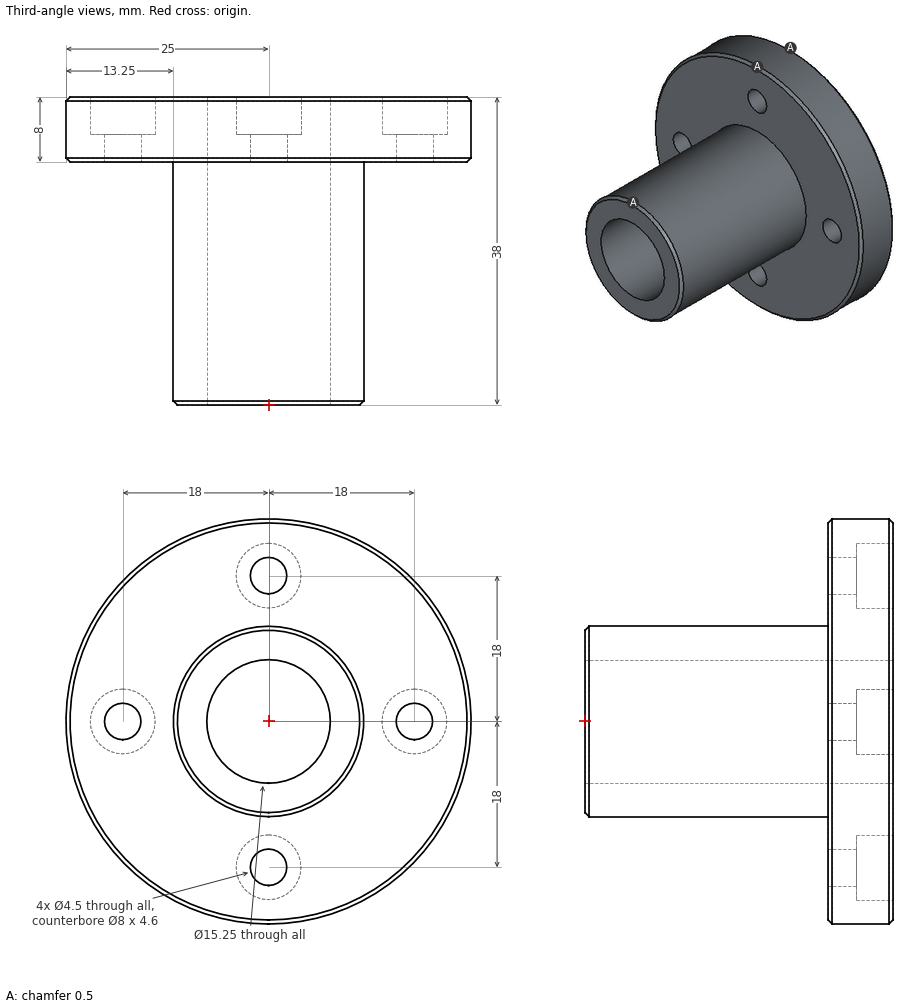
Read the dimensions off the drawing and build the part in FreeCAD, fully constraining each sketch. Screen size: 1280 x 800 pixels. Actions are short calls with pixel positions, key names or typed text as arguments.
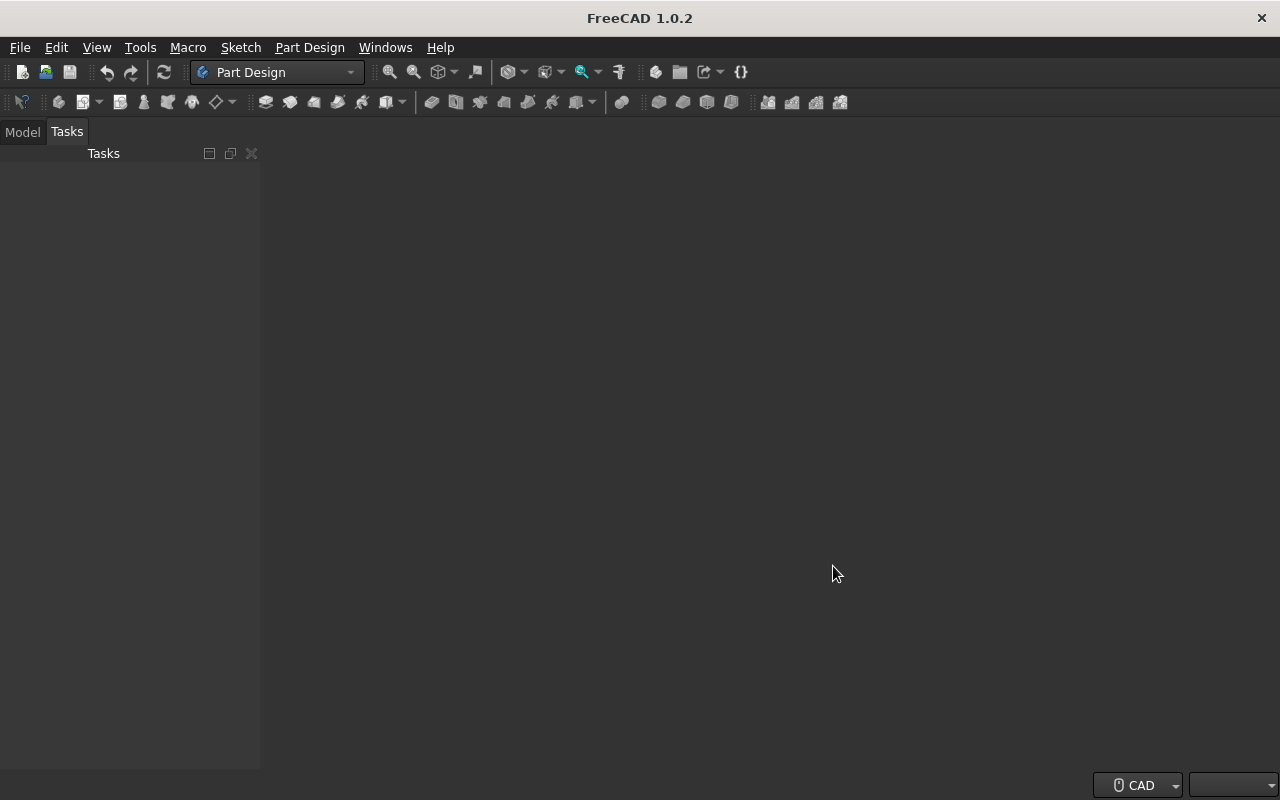
key(ctrl+n)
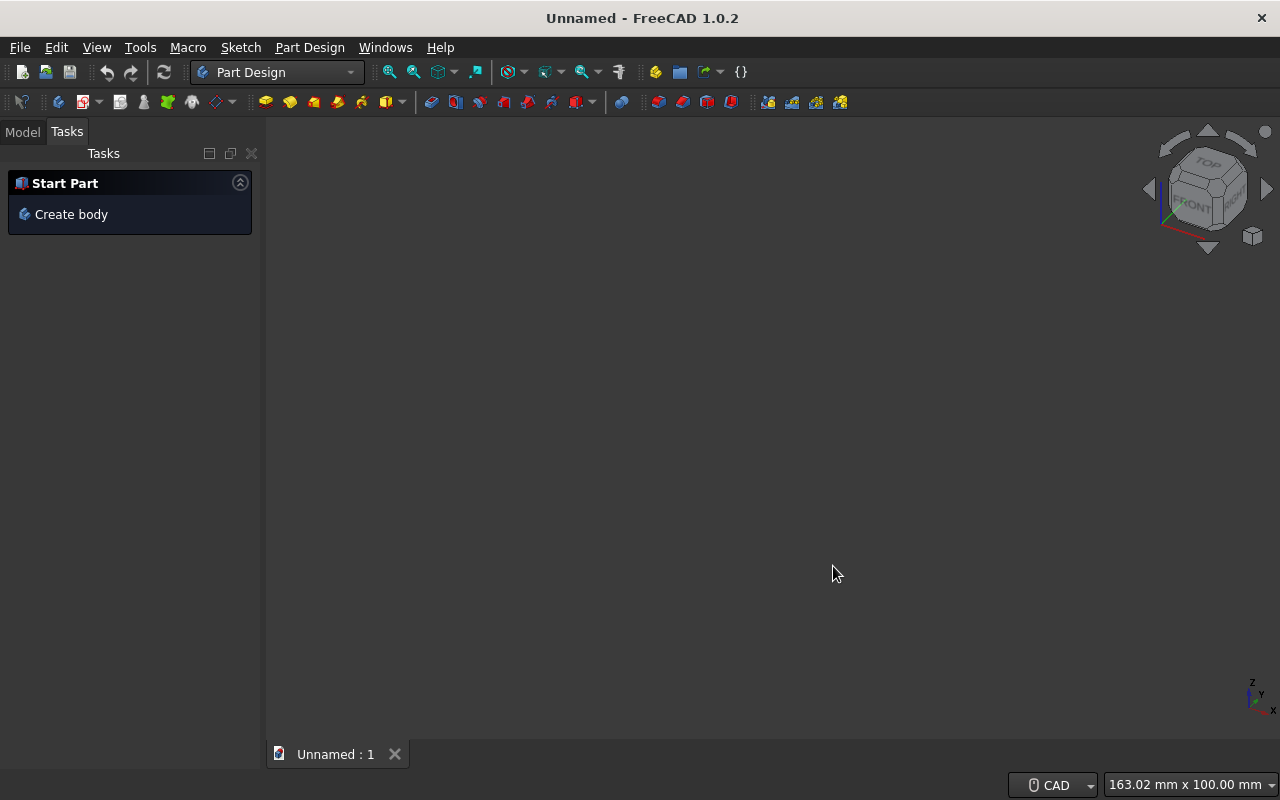
click(84, 102)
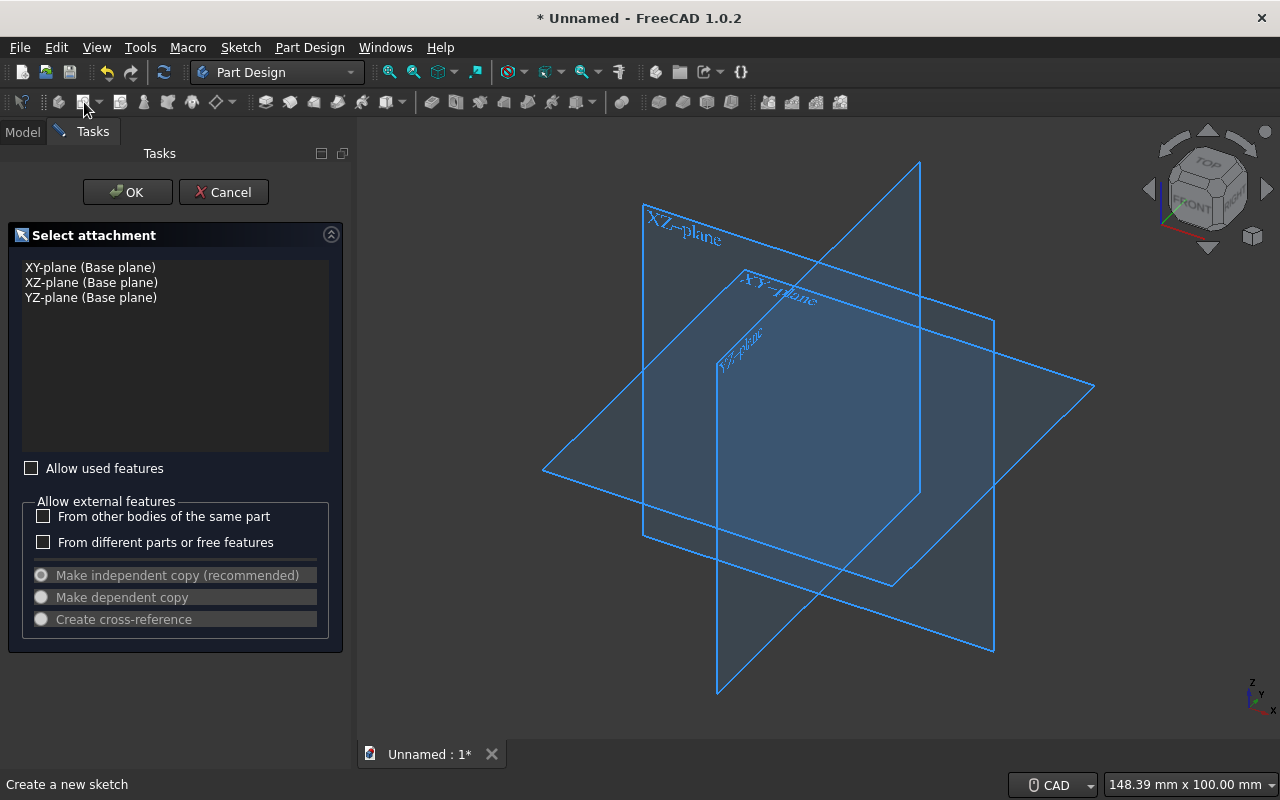
click(82, 268)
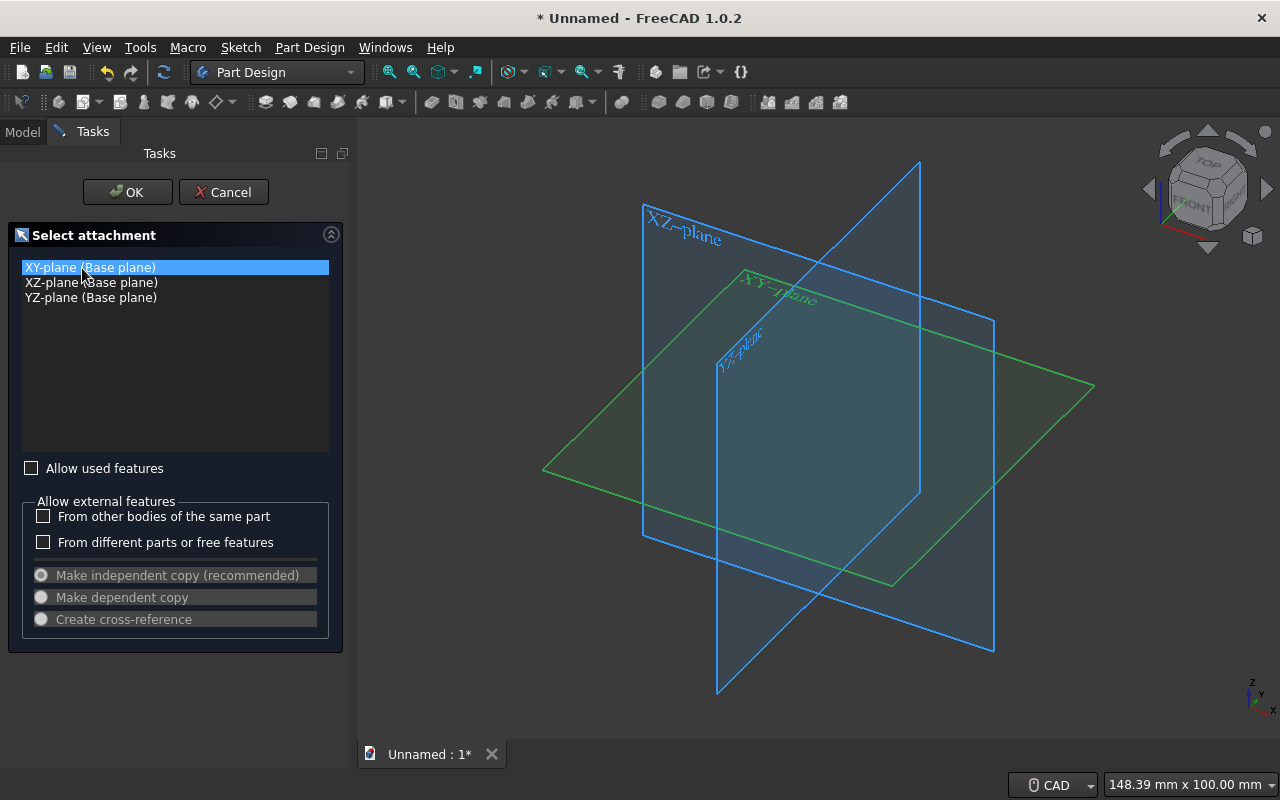
click(128, 192)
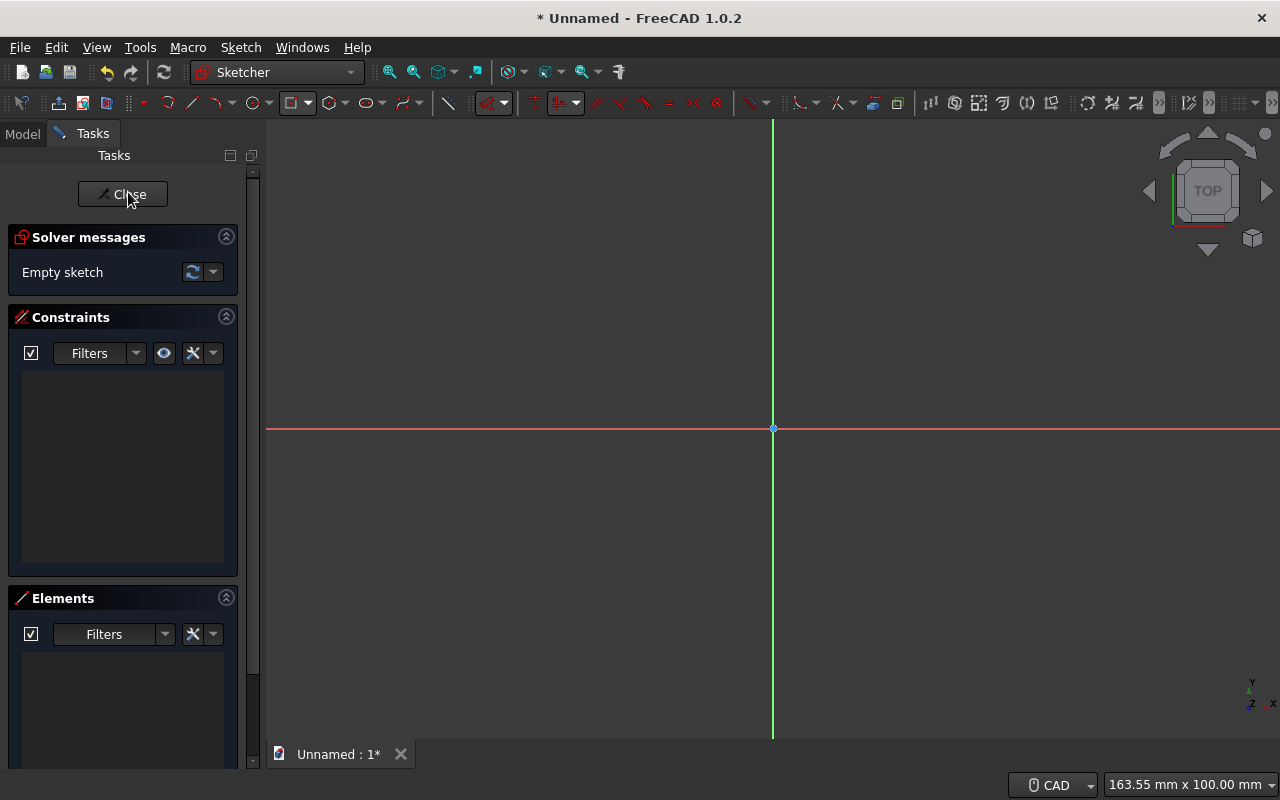
scroll(685, 168, up, 3)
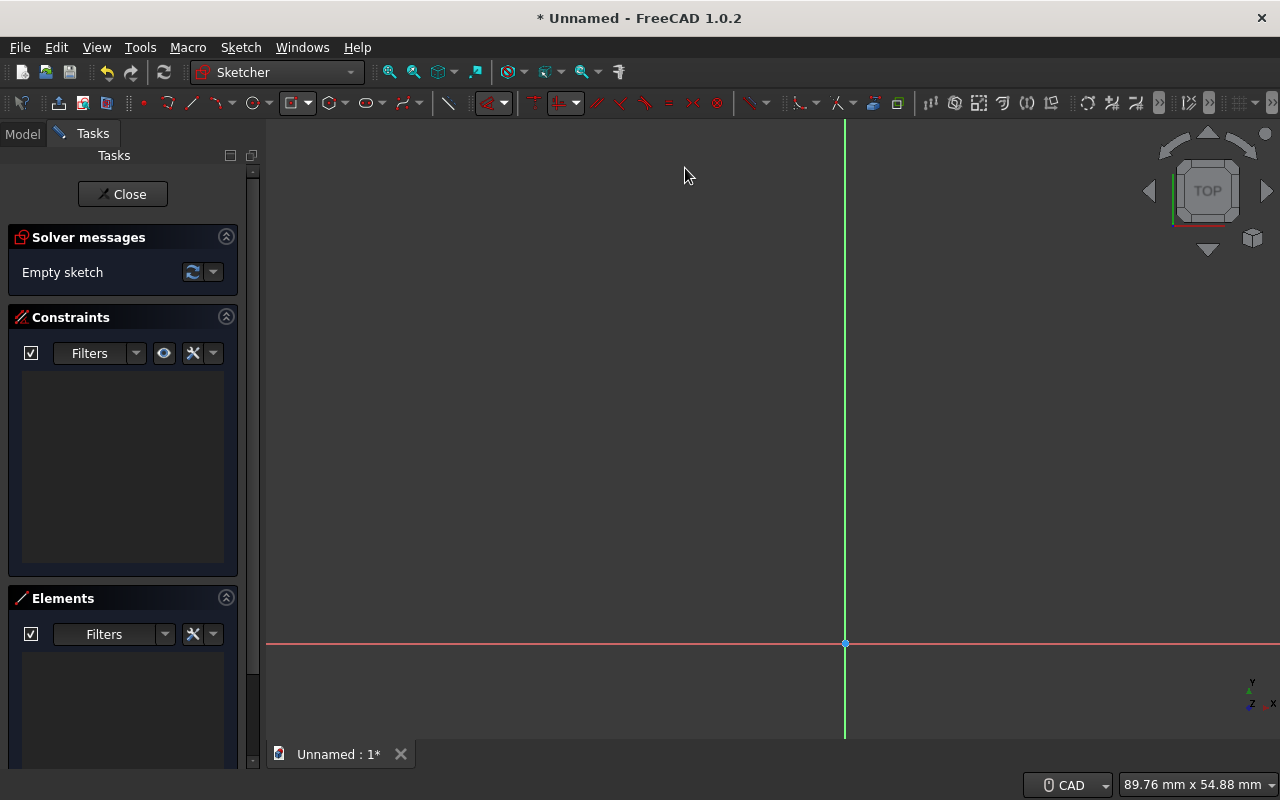
click(168, 104)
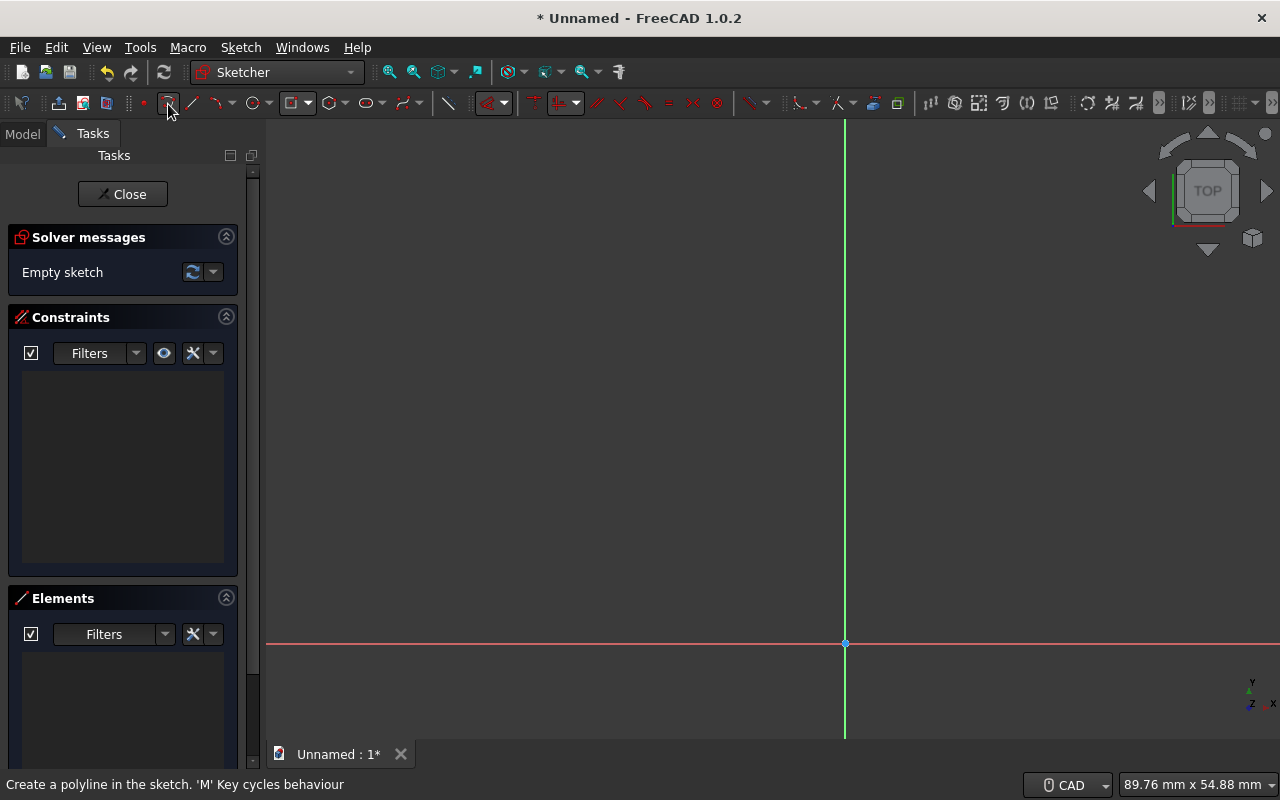
click(845, 644)
click(836, 214)
click(563, 214)
click(563, 305)
click(712, 305)
click(712, 635)
click(845, 644)
key(Escape)
key(Escape)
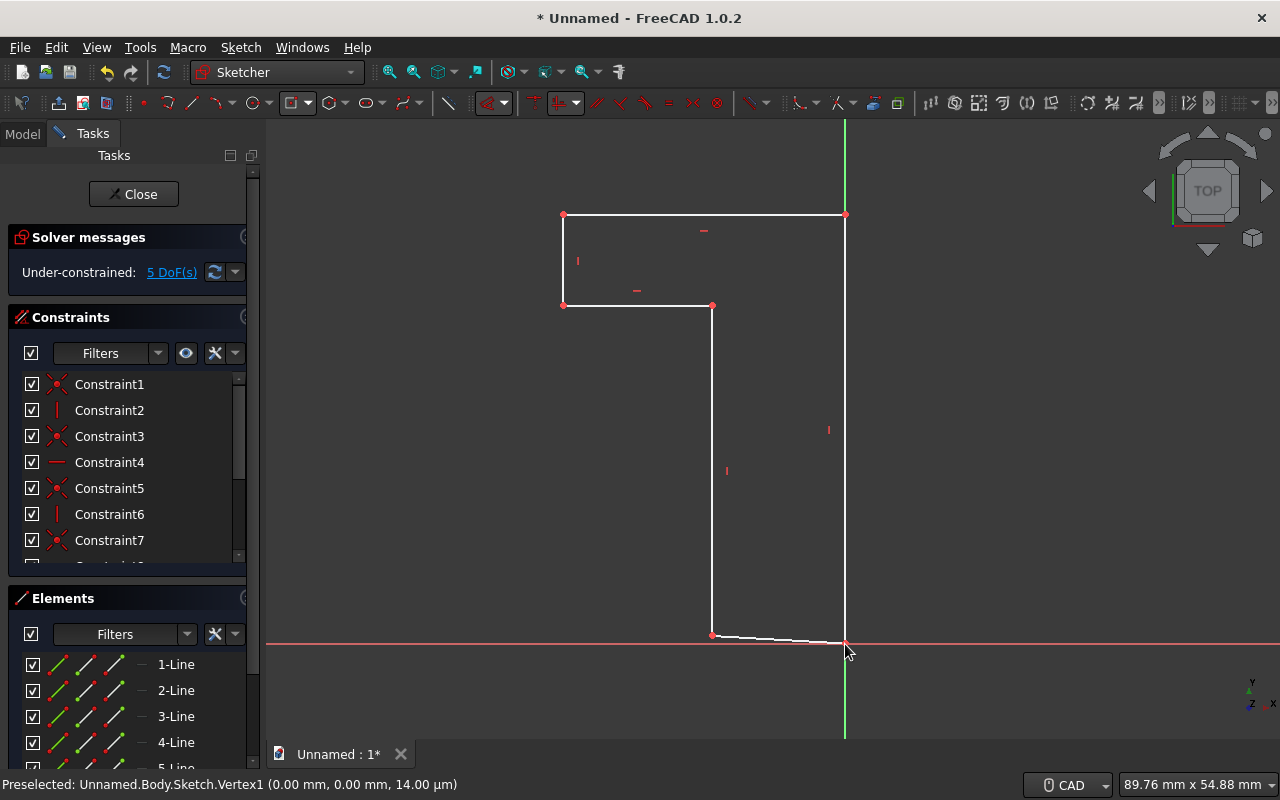
click(805, 641)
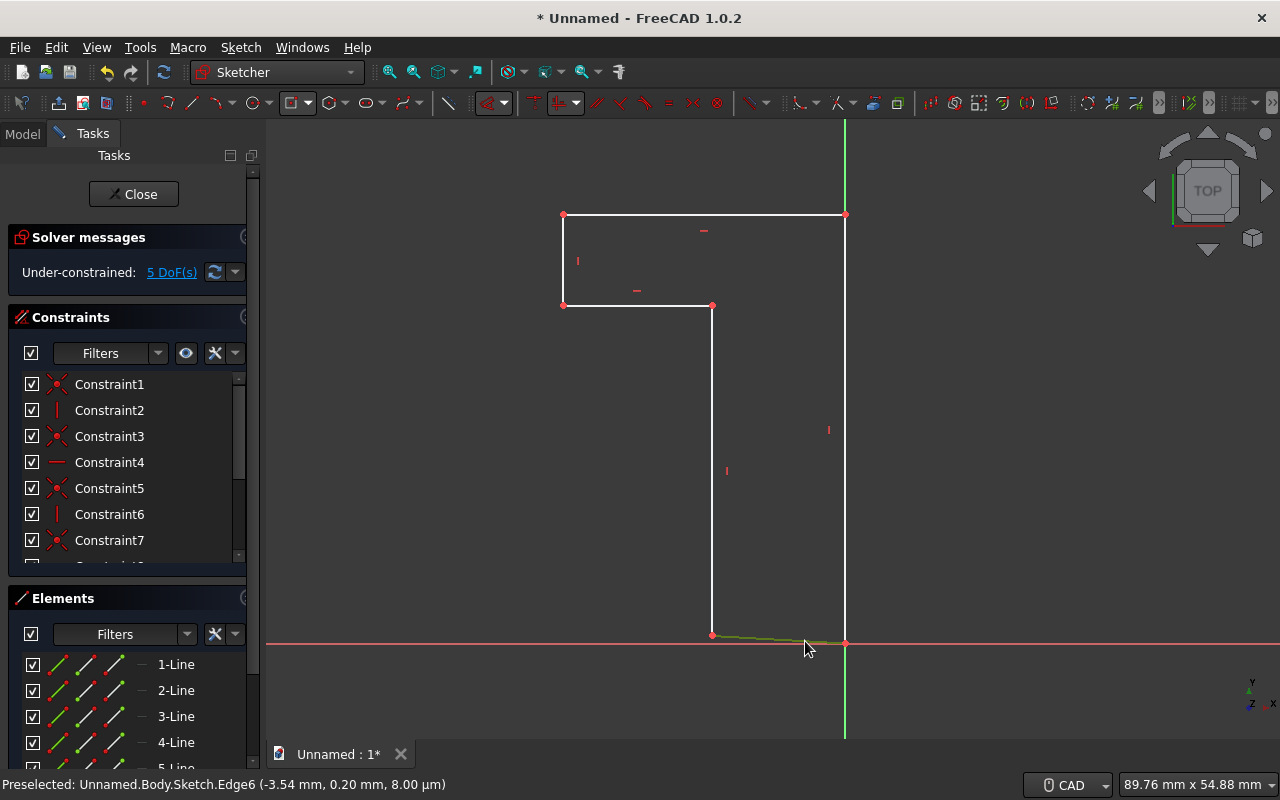
click(578, 104)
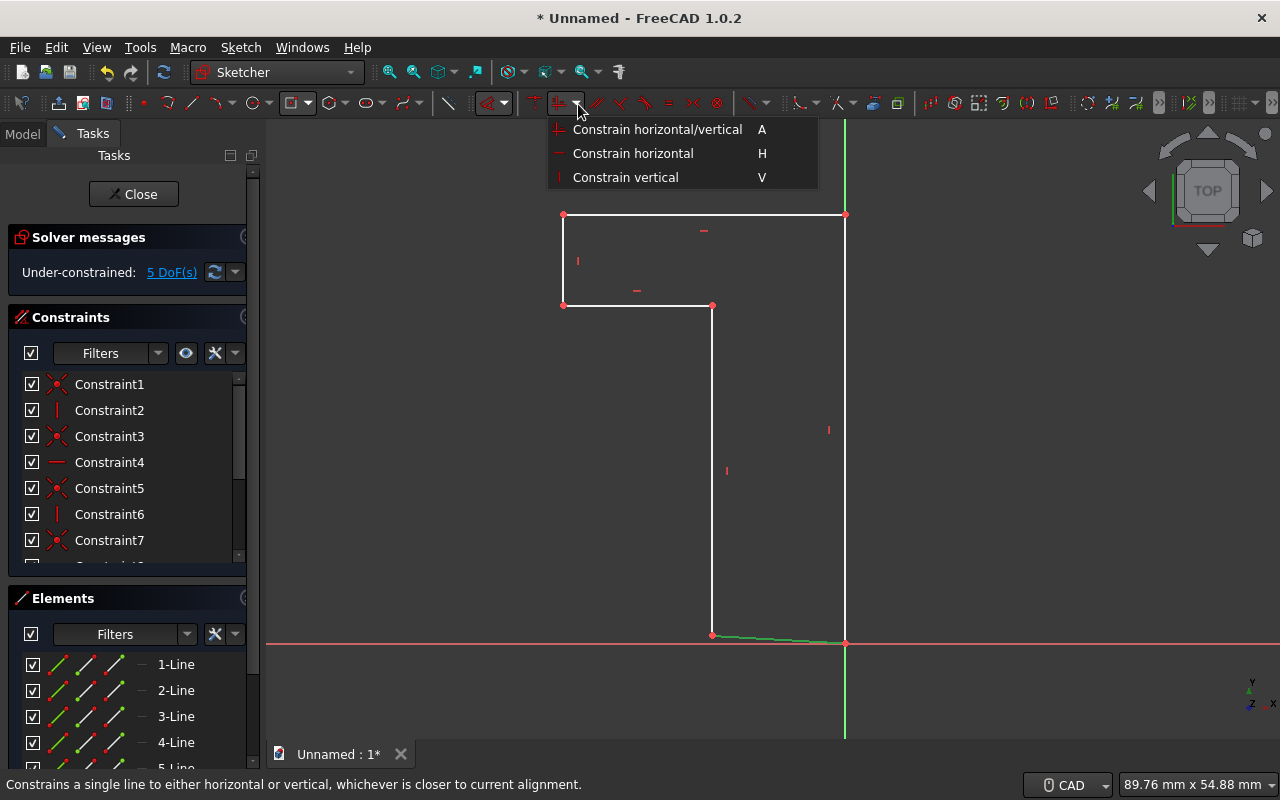
click(683, 153)